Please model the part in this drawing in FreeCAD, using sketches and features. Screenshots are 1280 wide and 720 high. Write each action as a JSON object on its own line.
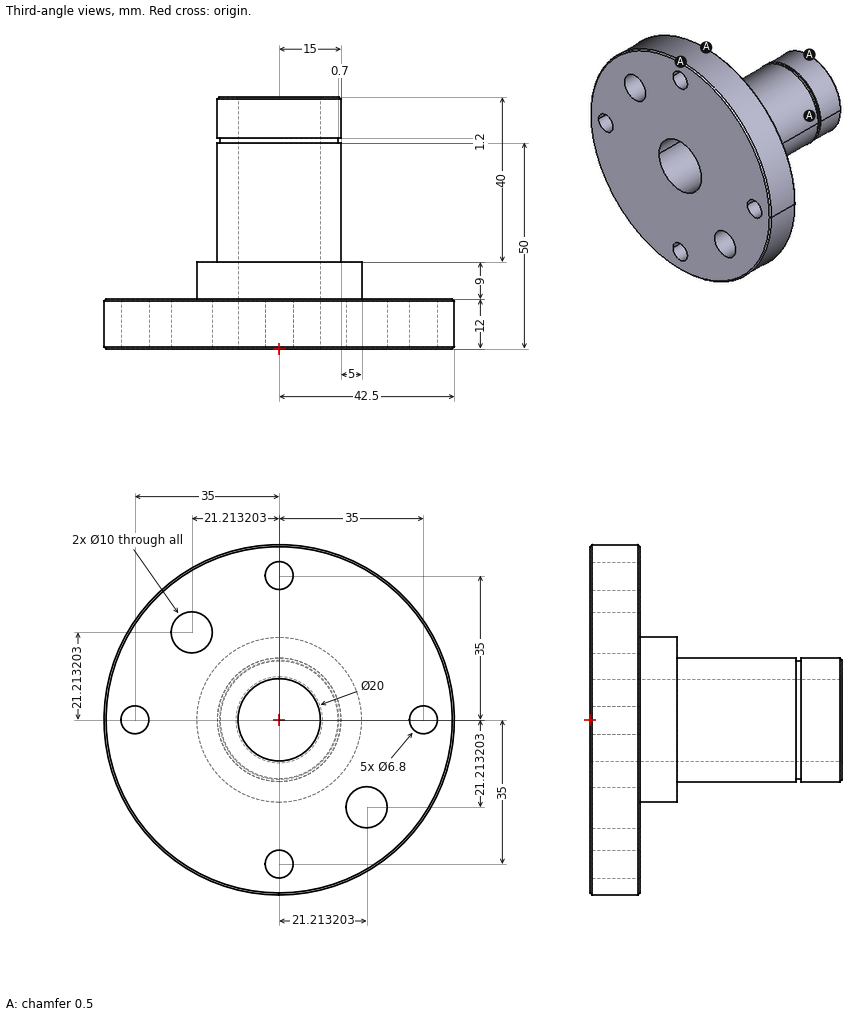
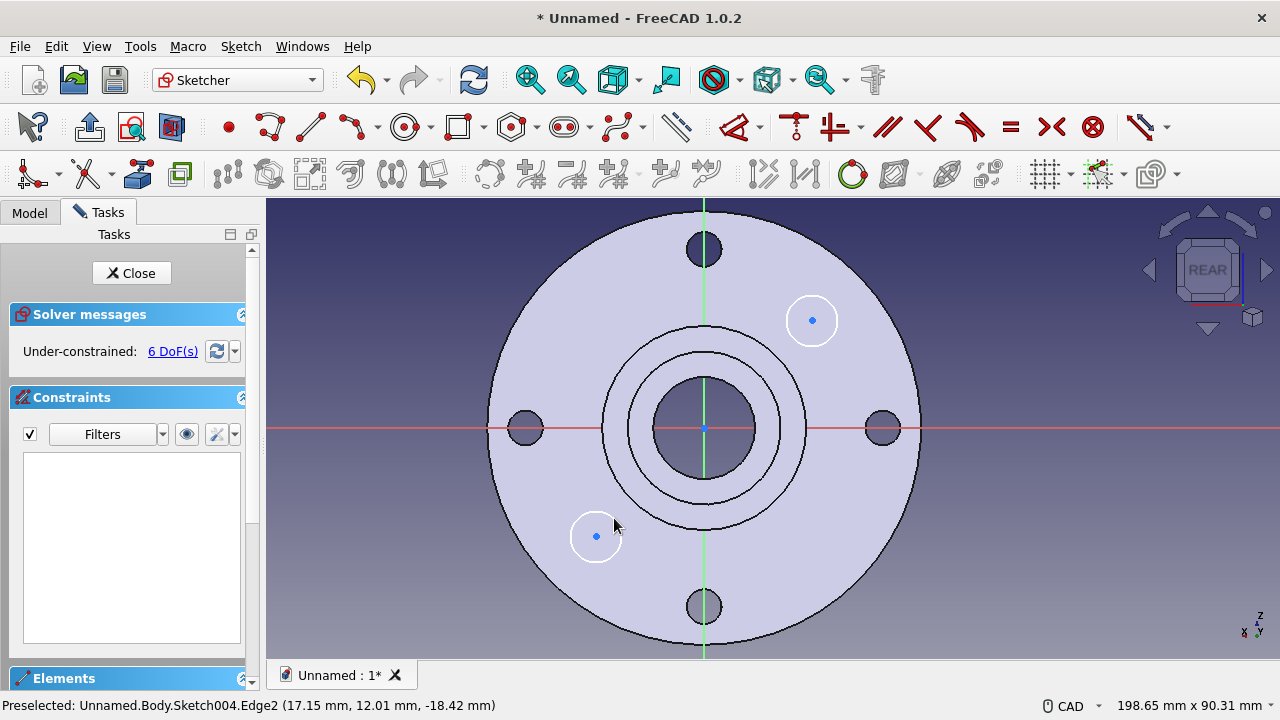
{"action": "left_click", "coordinate": [830, 303]}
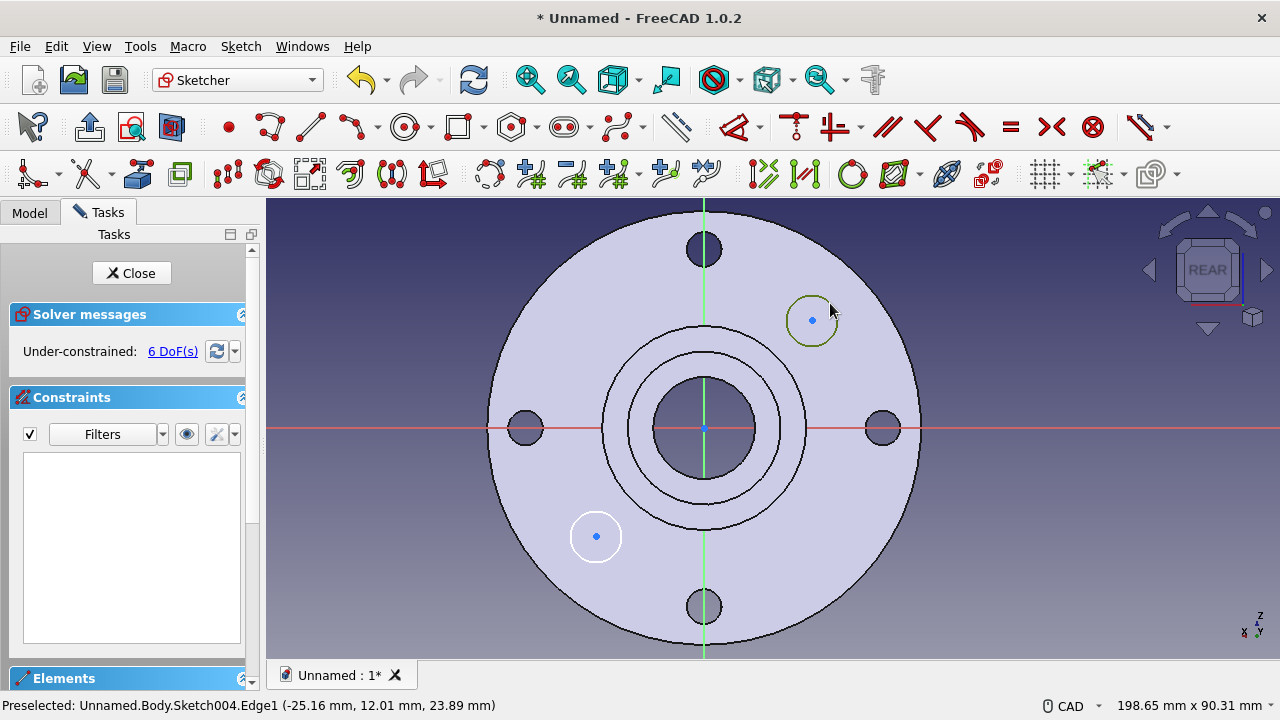
{"action": "left_click", "coordinate": [614, 519]}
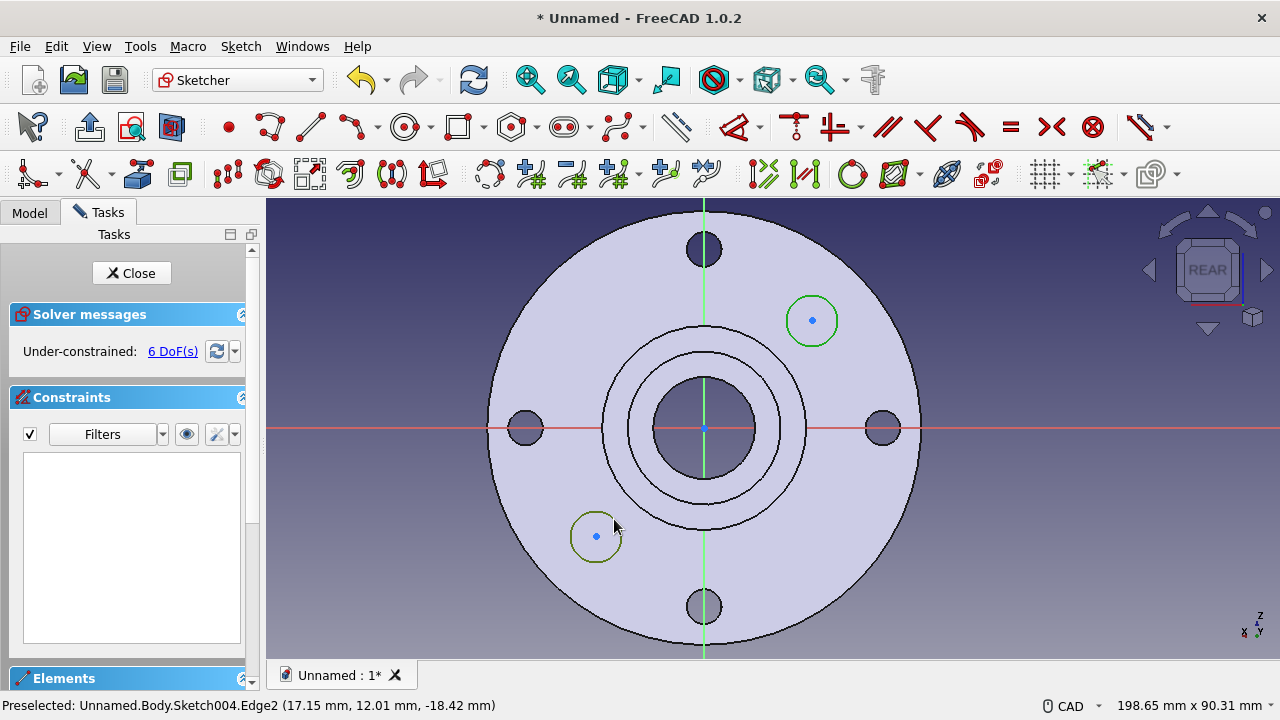
{"action": "left_click", "coordinate": [1011, 128]}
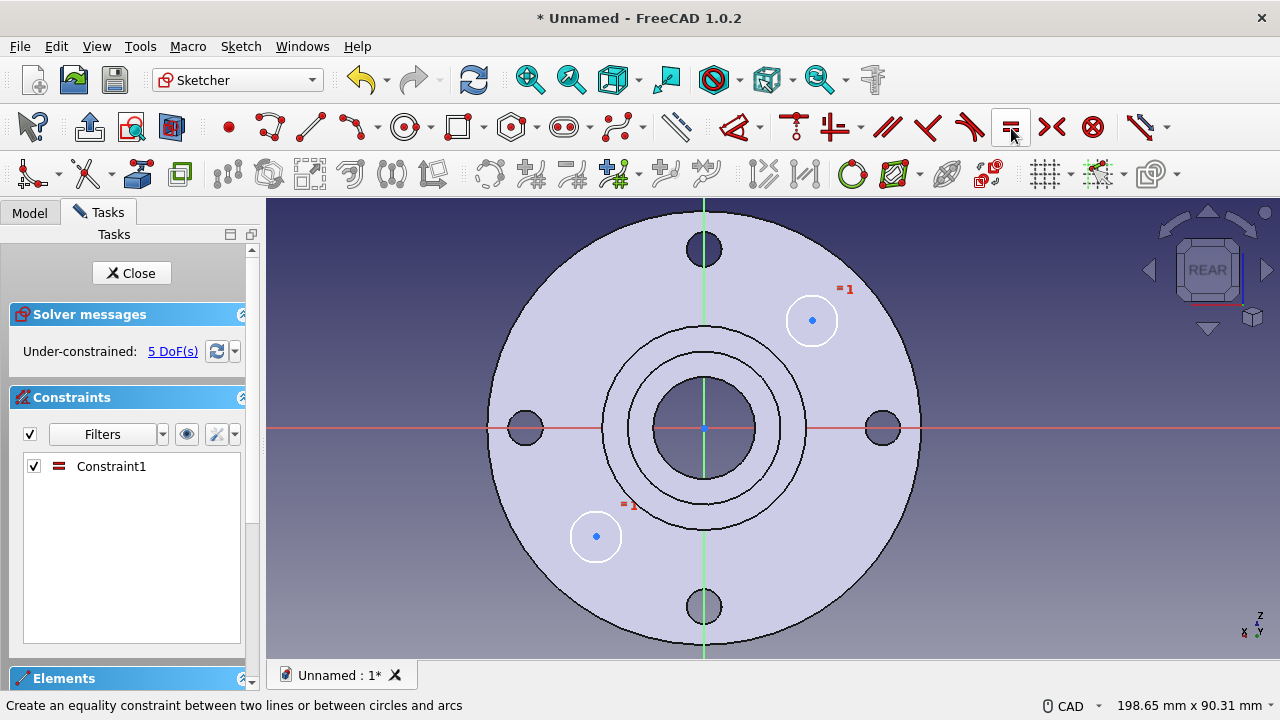
{"action": "left_click", "coordinate": [734, 128]}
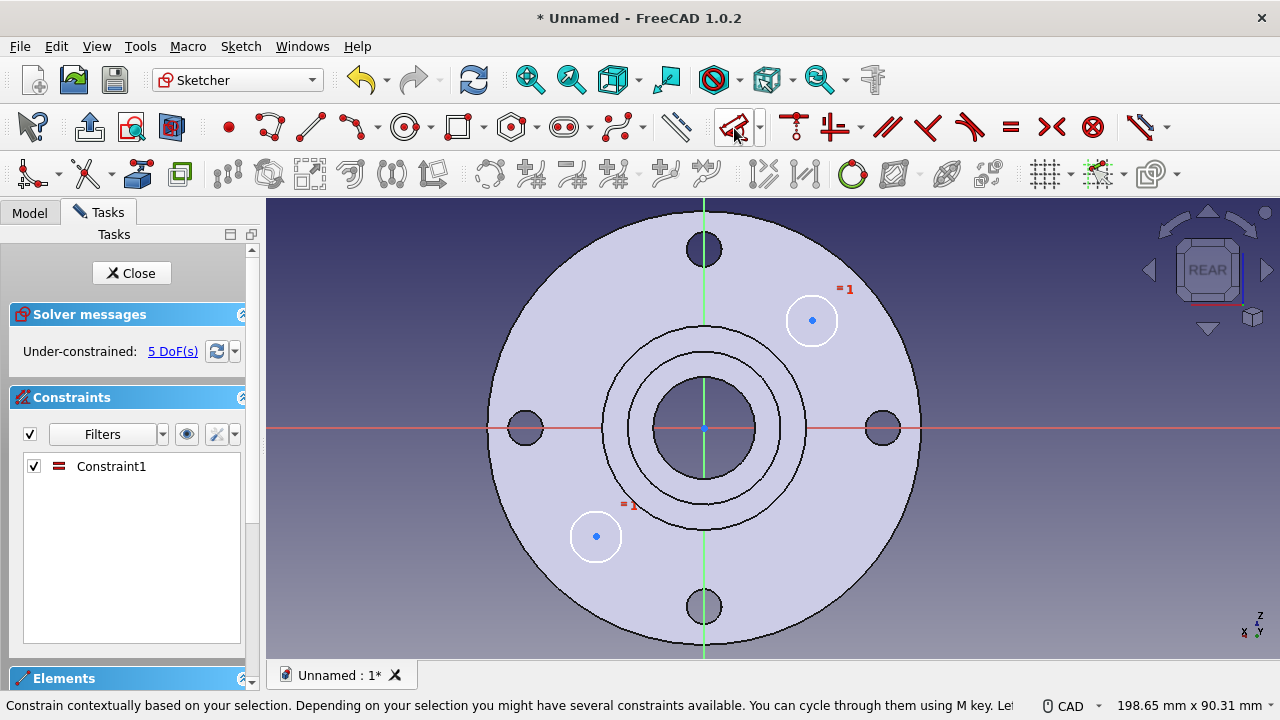
{"action": "left_click", "coordinate": [830, 303]}
{"action": "left_click", "coordinate": [853, 280]}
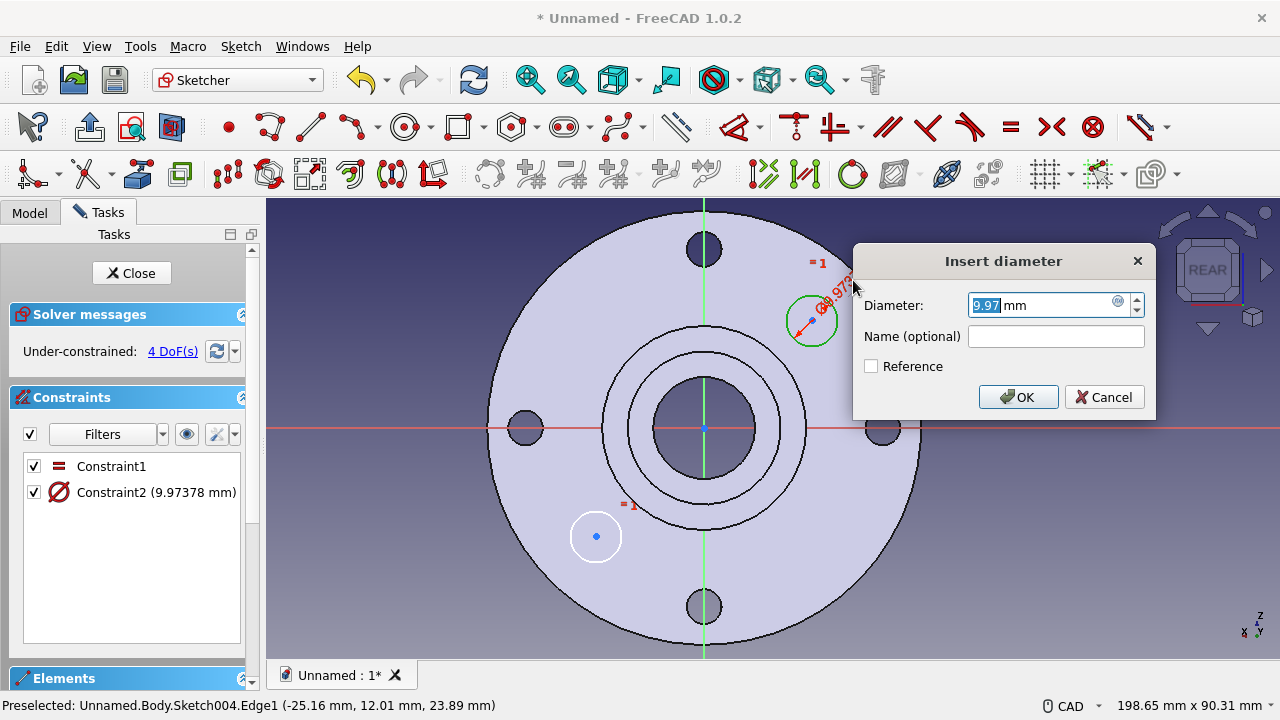
{"action": "type", "text": "10"}
{"action": "key", "text": "Return"}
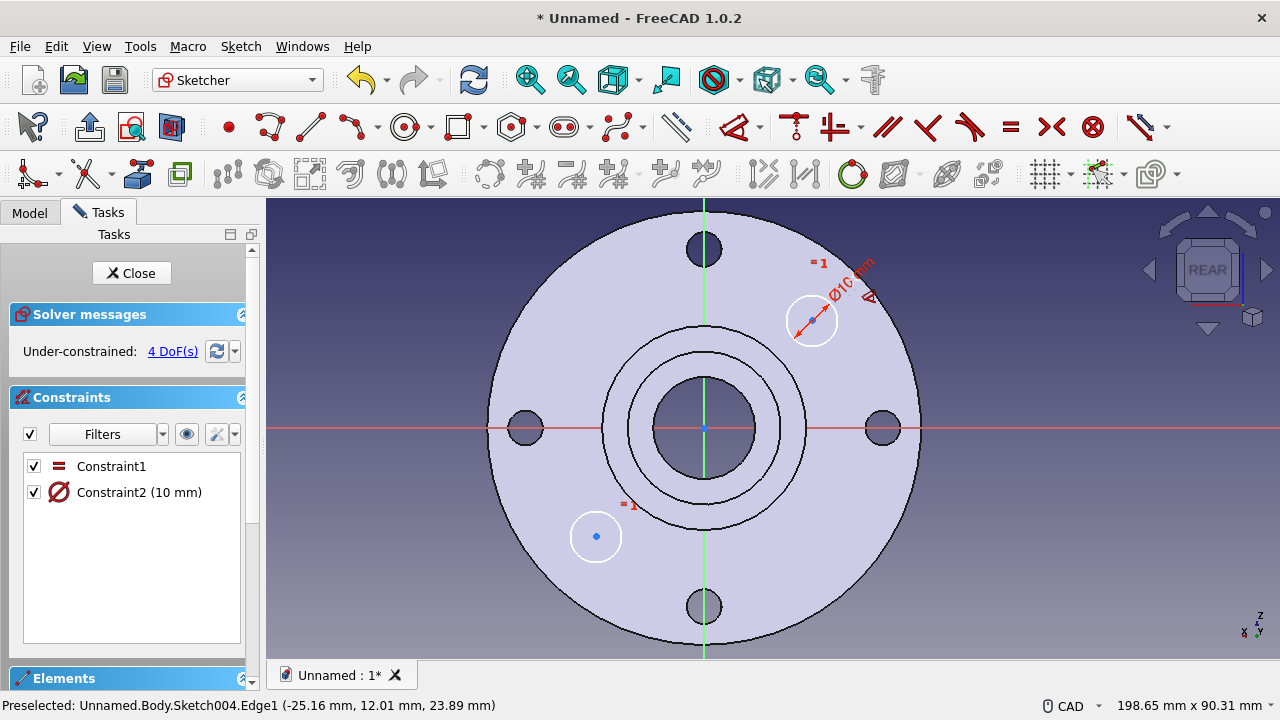
{"action": "left_click", "coordinate": [812, 321]}
{"action": "left_click", "coordinate": [758, 287]}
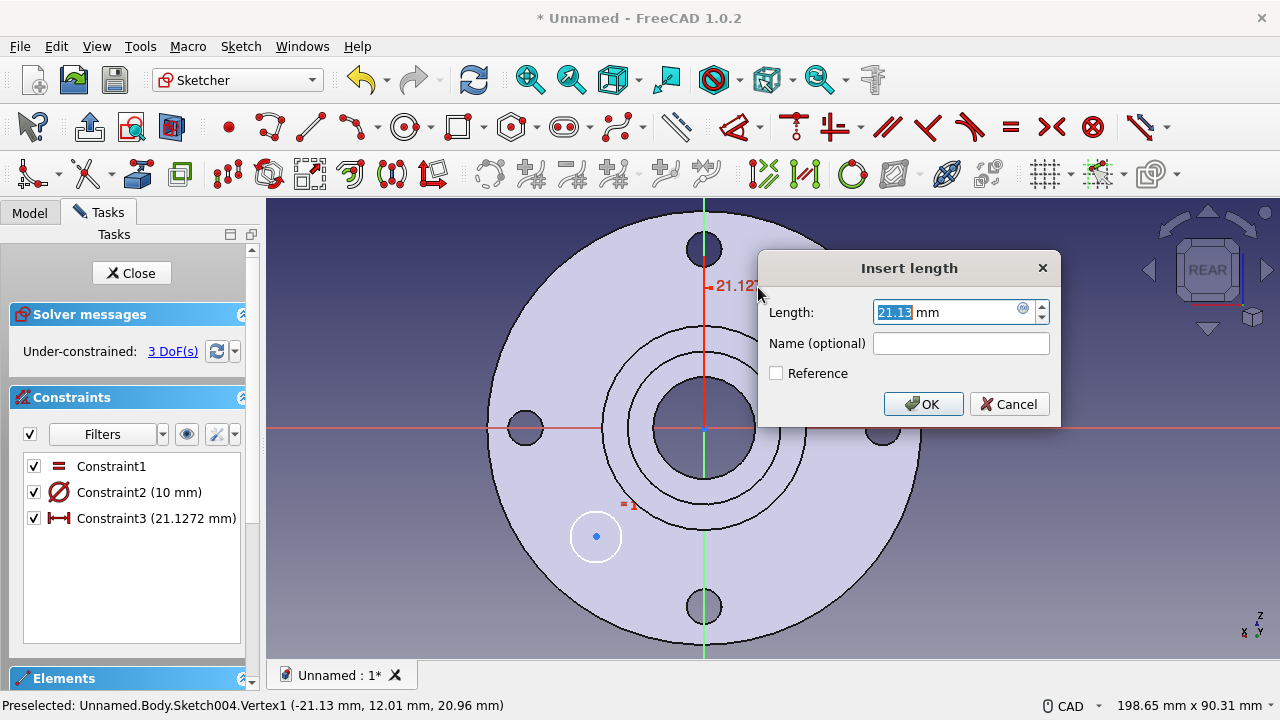
{"action": "type", "text": "21.213203"}
{"action": "key", "text": "Return"}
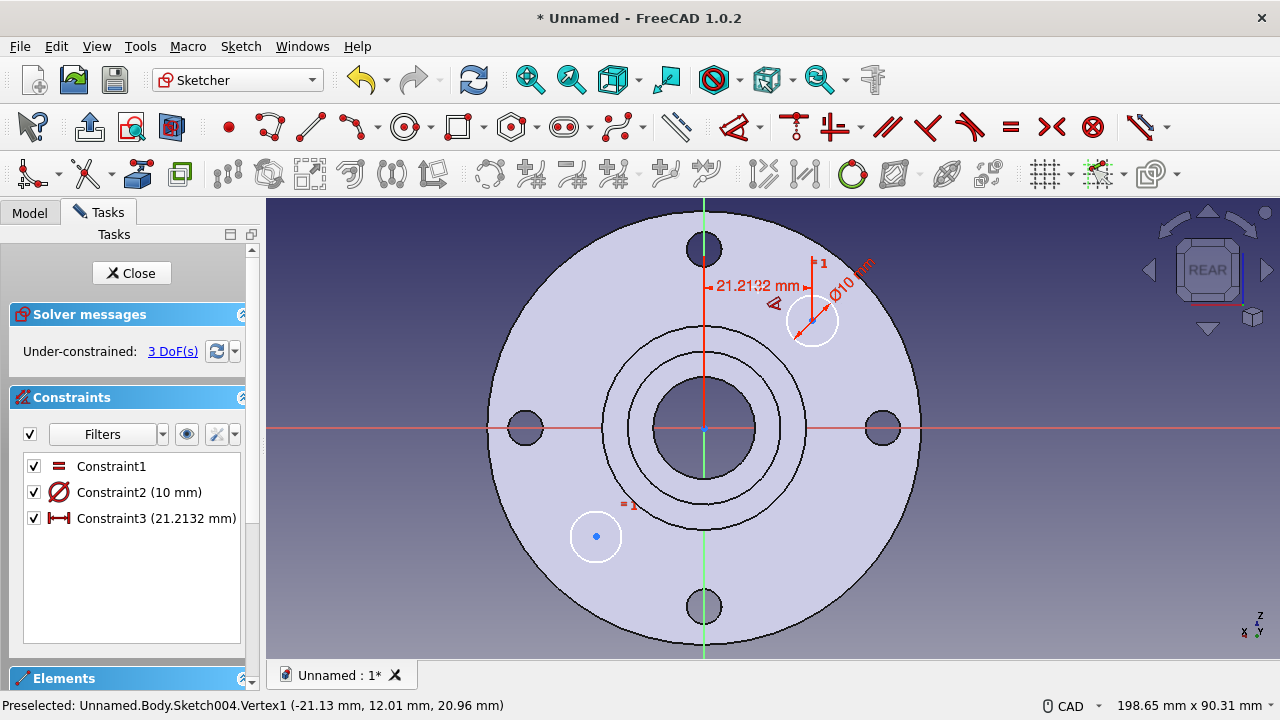
{"action": "left_click", "coordinate": [812, 321]}
{"action": "left_click", "coordinate": [846, 375]}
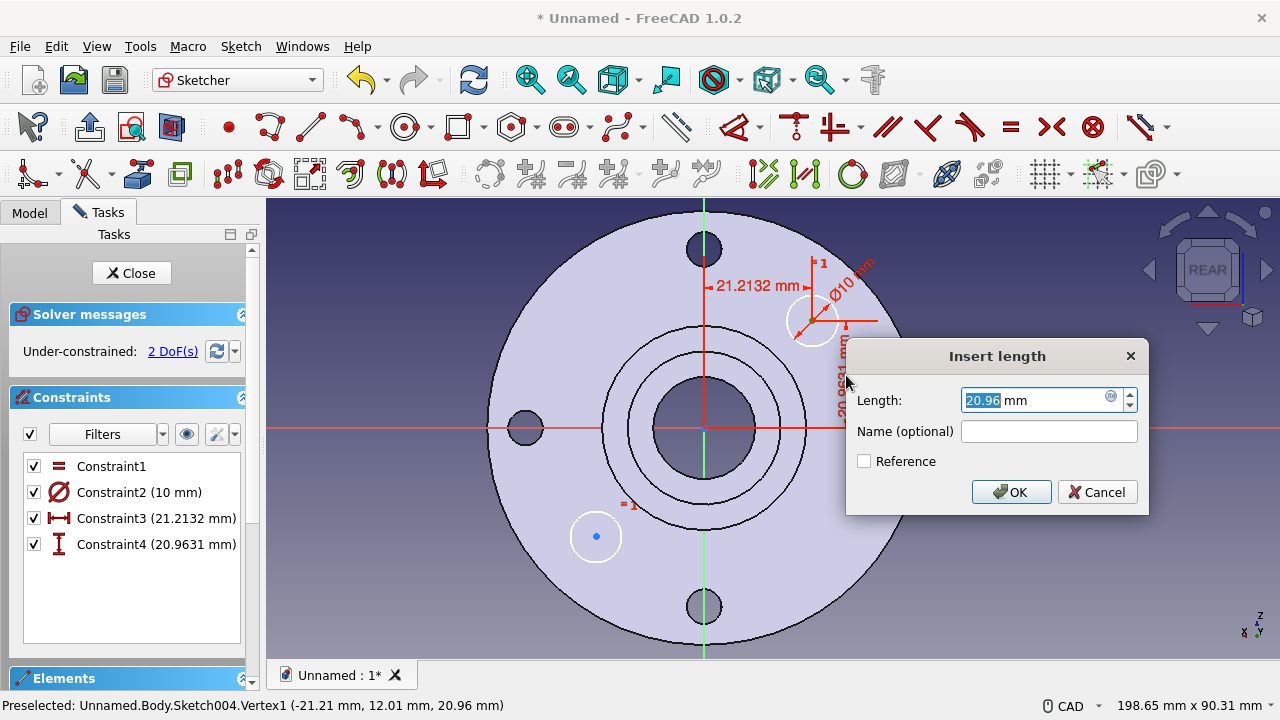
{"action": "type", "text": "21.213203"}
{"action": "key", "text": "Return"}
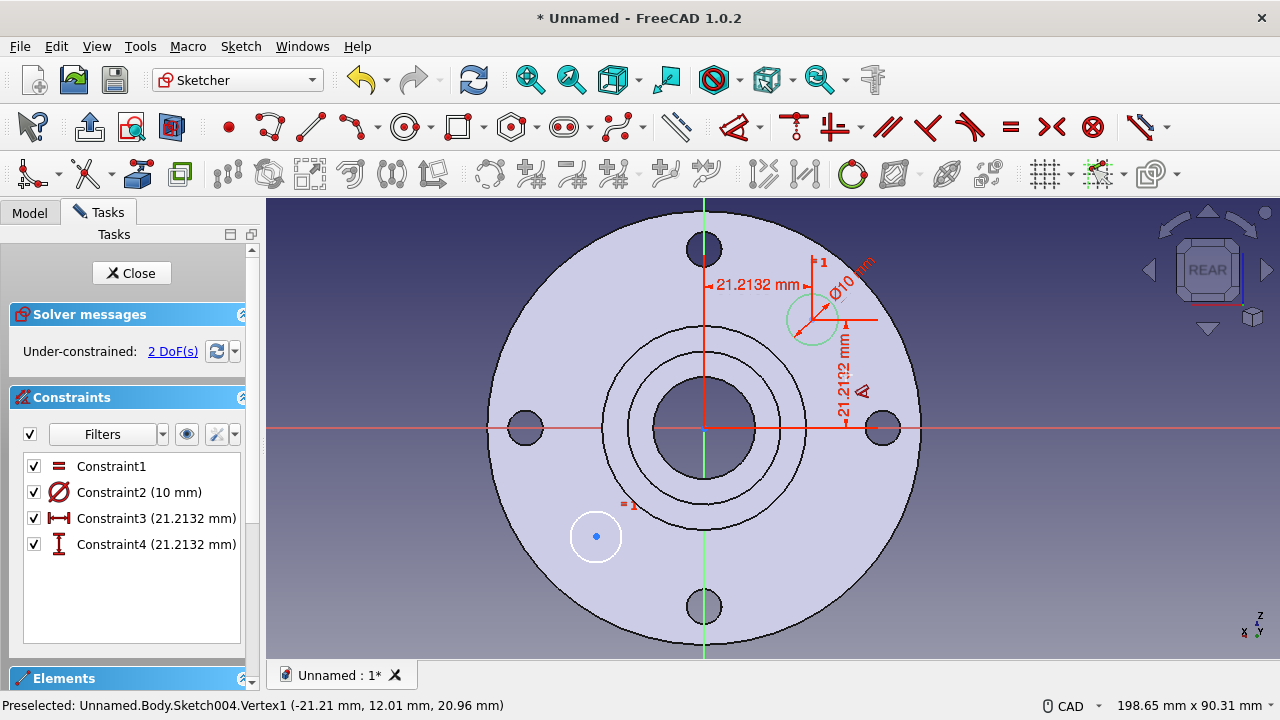
{"action": "left_click", "coordinate": [596, 537]}
{"action": "left_click", "coordinate": [650, 571]}